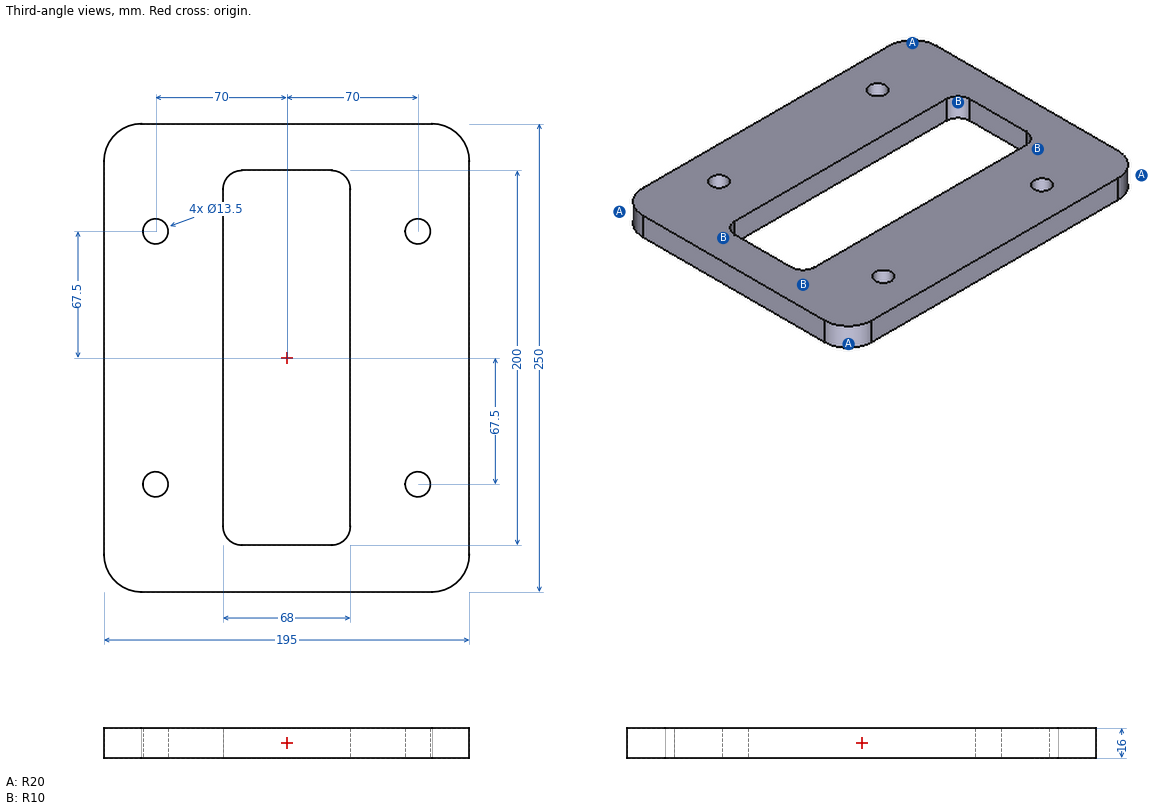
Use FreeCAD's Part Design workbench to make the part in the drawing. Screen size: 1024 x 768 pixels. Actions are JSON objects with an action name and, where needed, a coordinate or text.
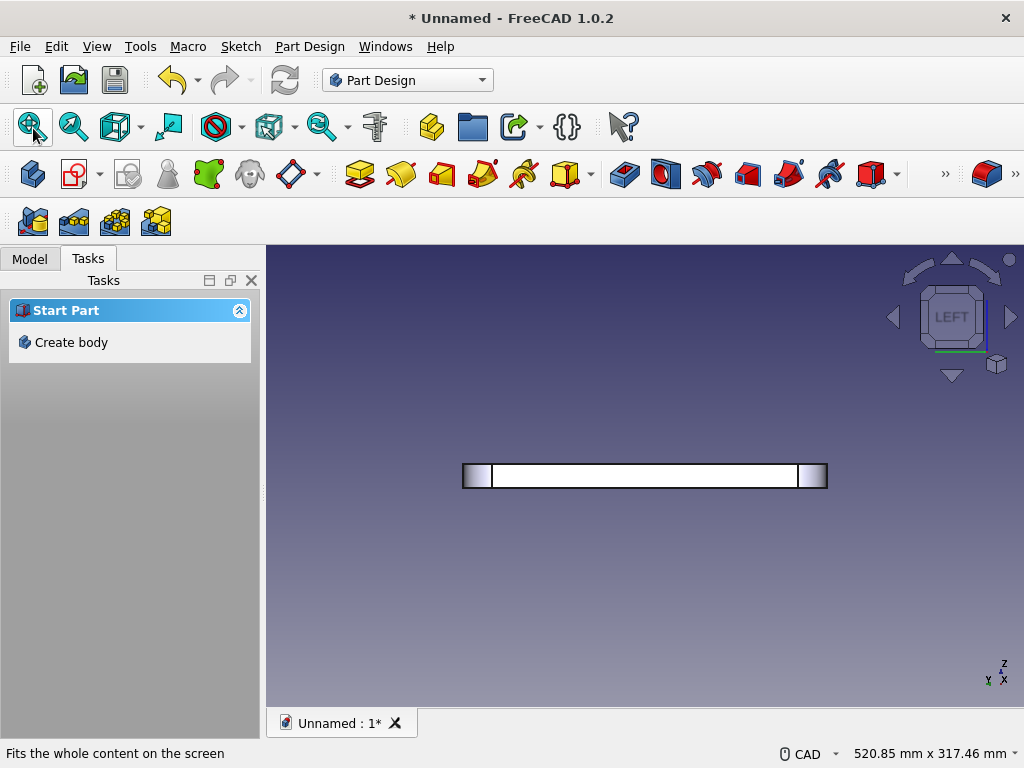
{"action": "key", "text": "v 3"}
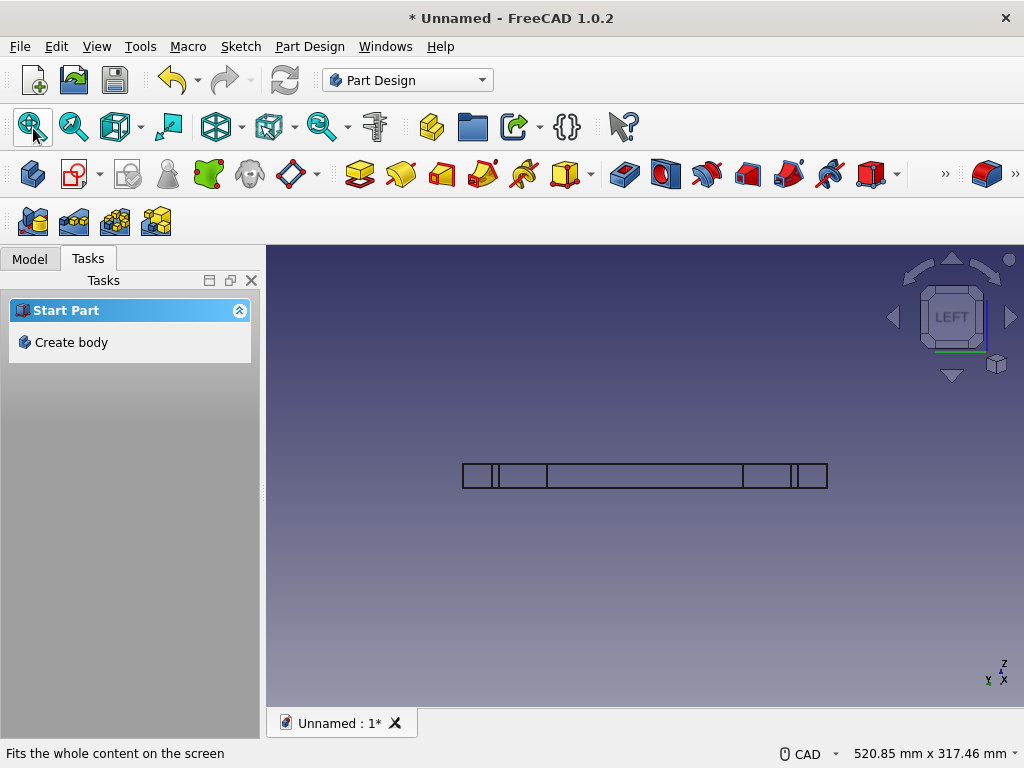
{"action": "key", "text": "0"}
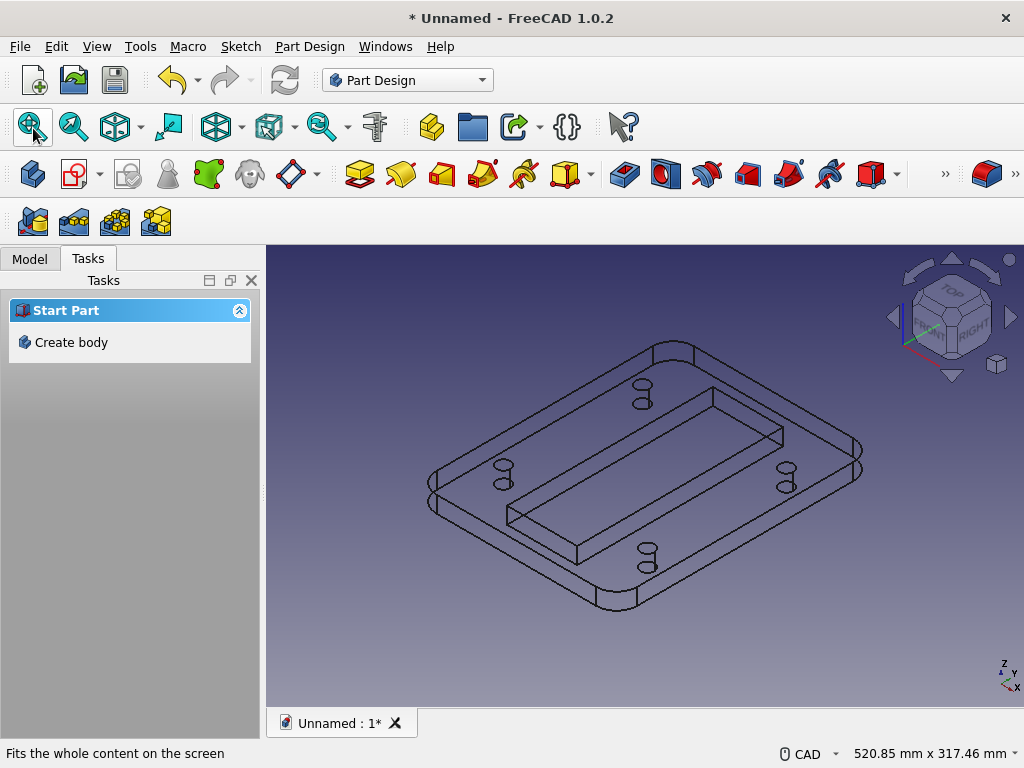
{"action": "left_click", "coordinate": [713, 395]}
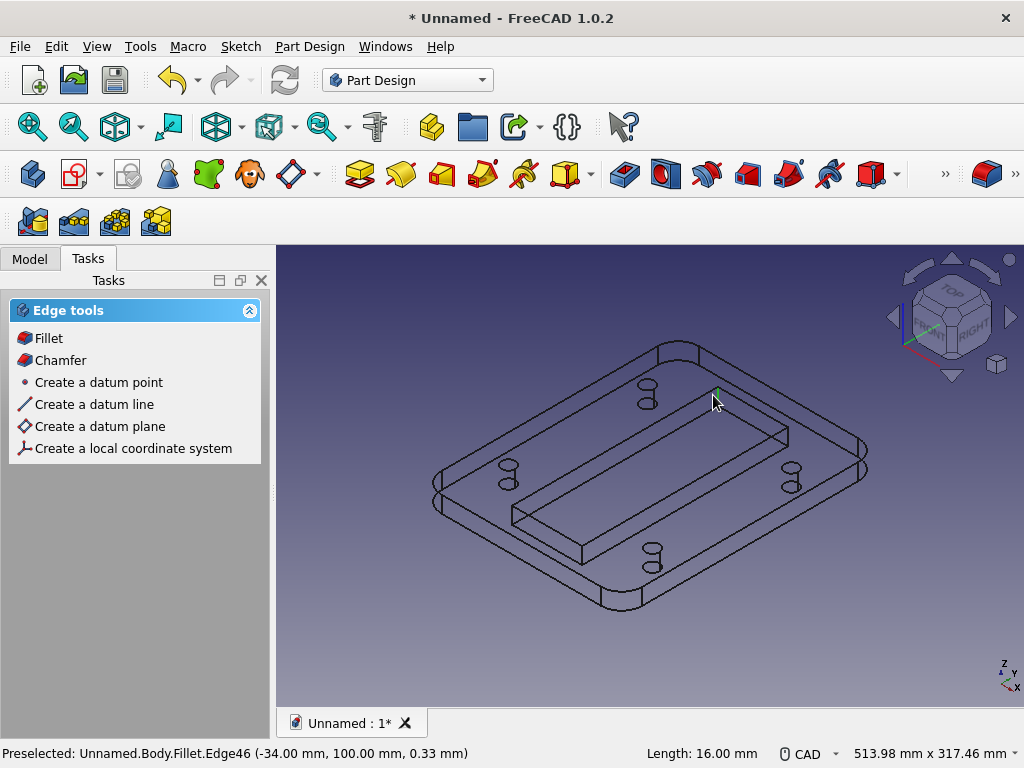
{"action": "left_click", "coordinate": [512, 514], "text": "ctrl"}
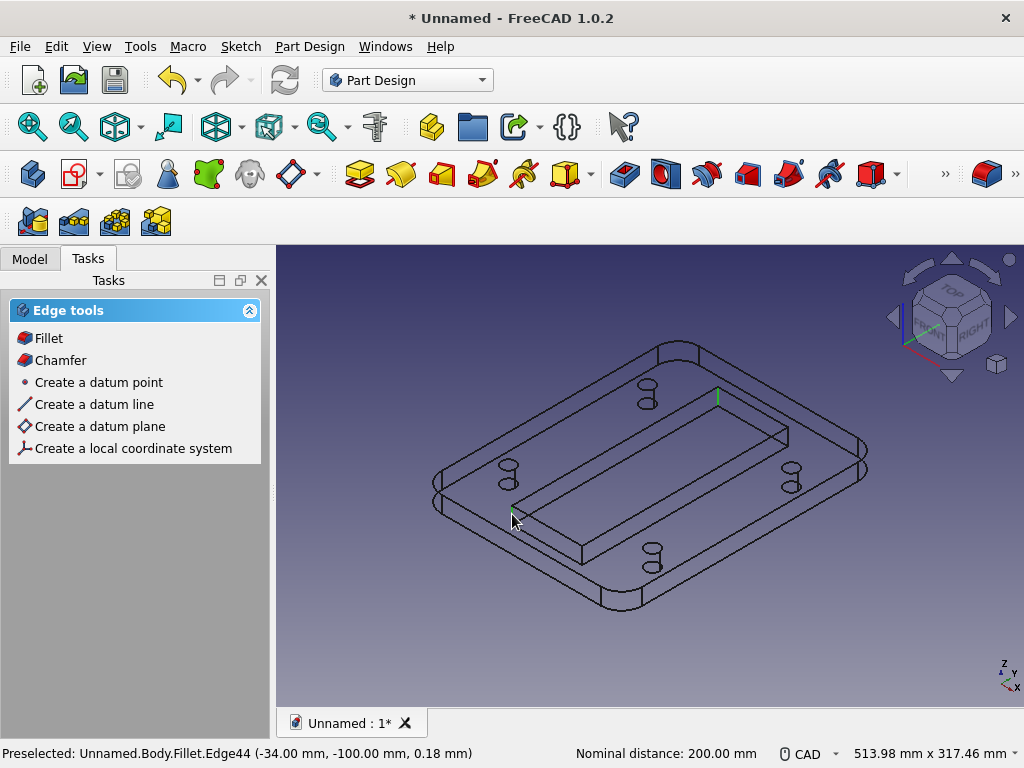
{"action": "left_click", "coordinate": [582, 555], "text": "ctrl"}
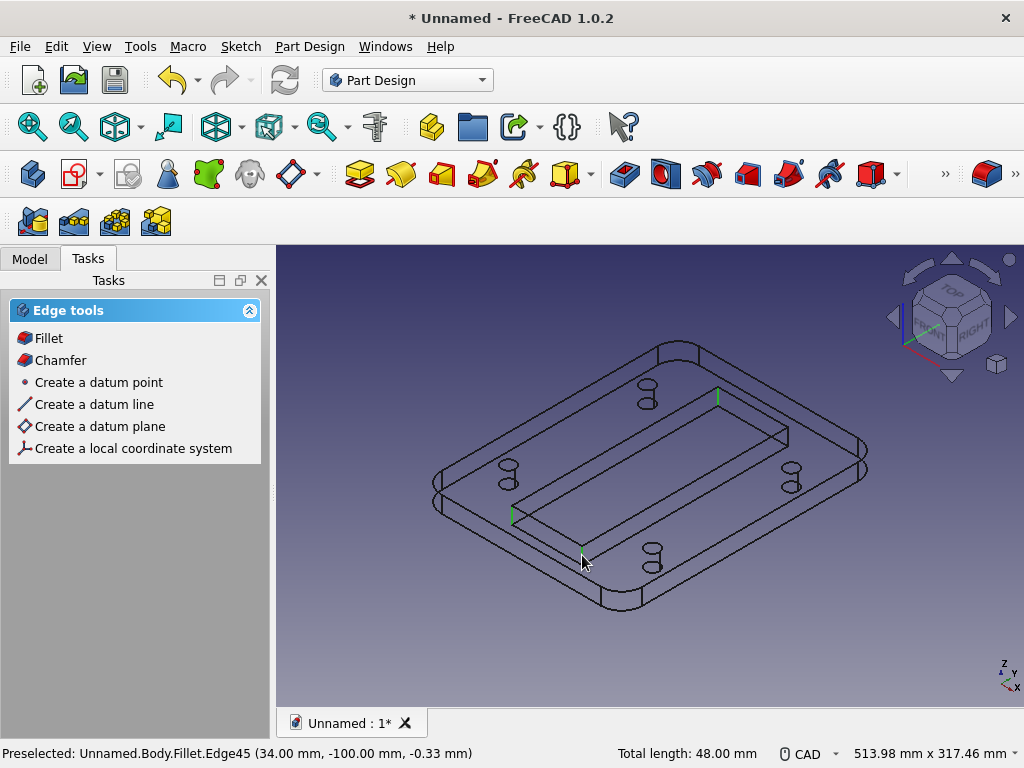
{"action": "left_click", "coordinate": [788, 436], "text": "ctrl"}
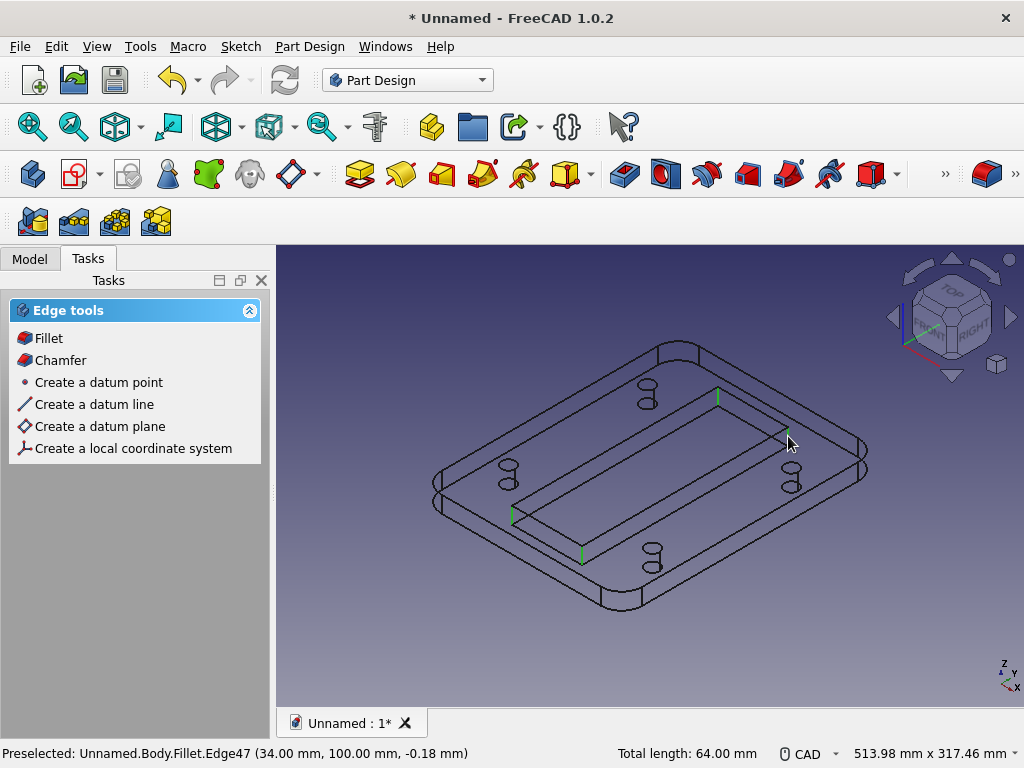
{"action": "key", "text": "v 1"}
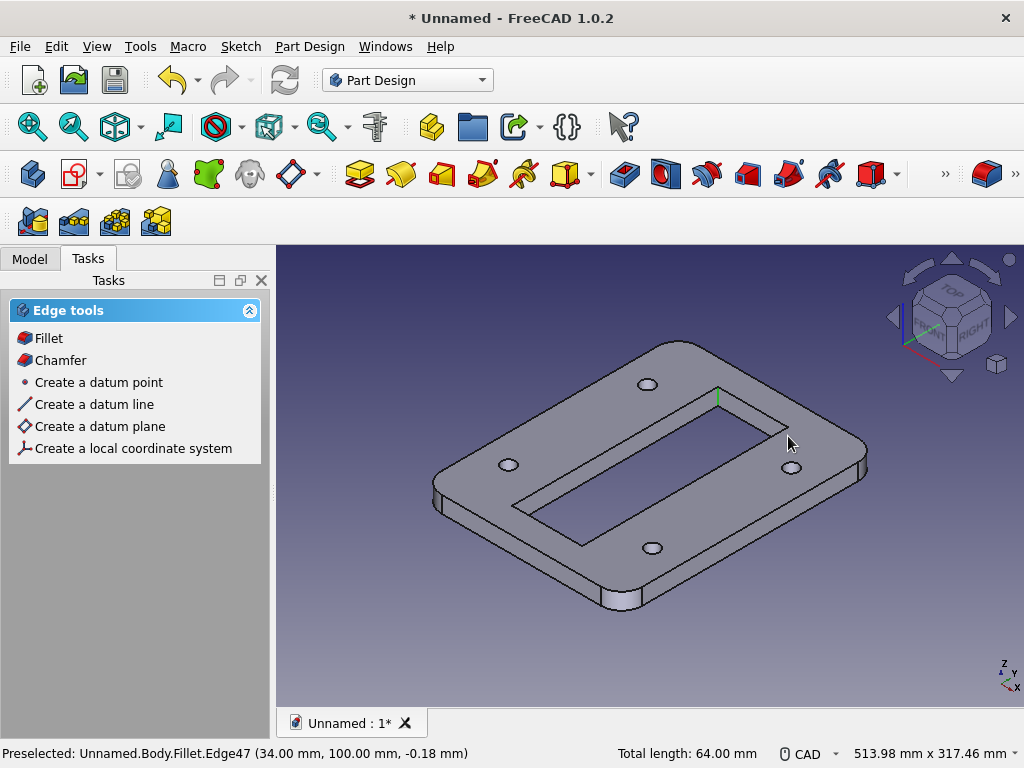
{"action": "left_click", "coordinate": [987, 174]}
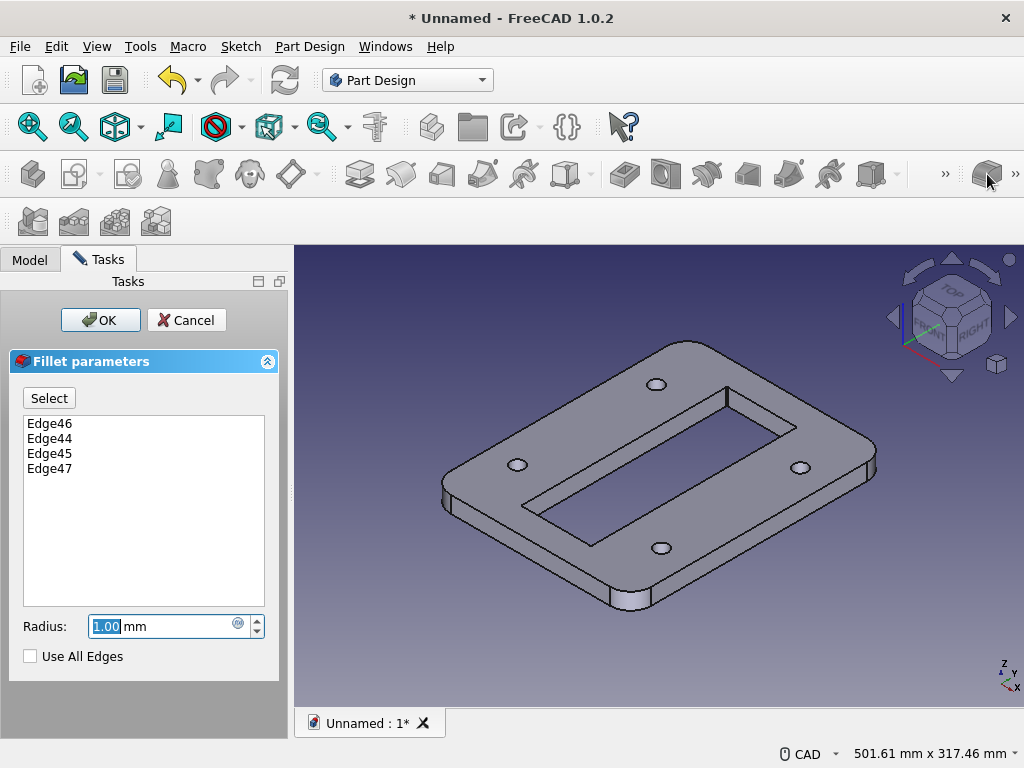
{"action": "type", "text": "10"}
{"action": "key", "text": "Tab"}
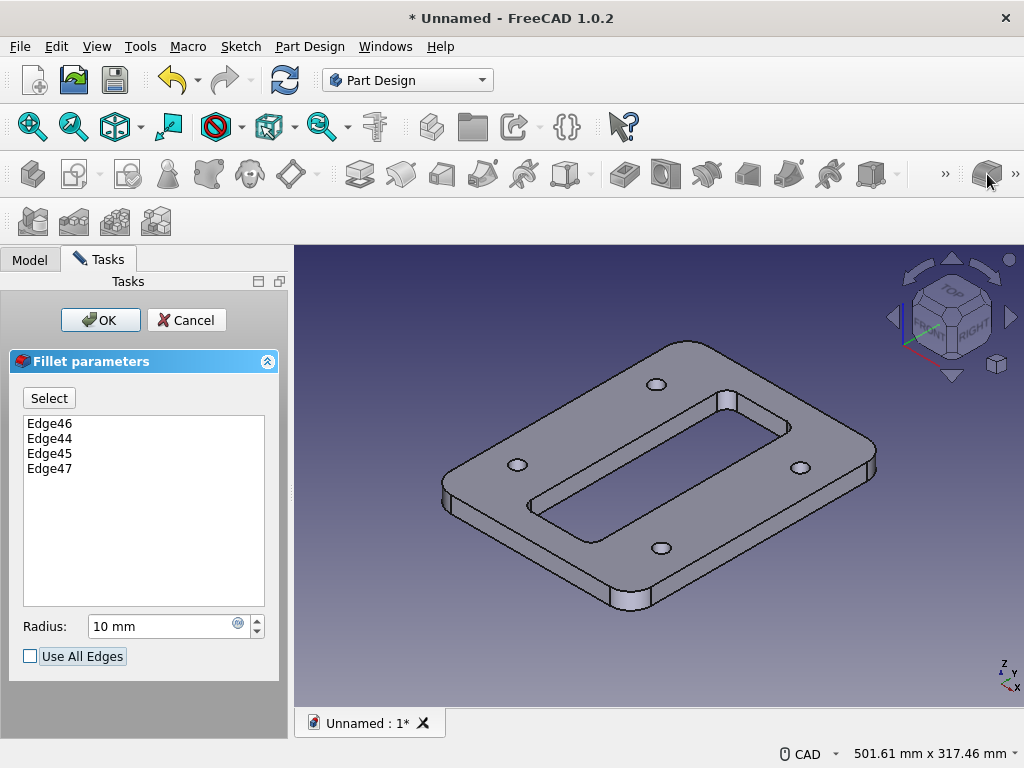
{"action": "left_click", "coordinate": [101, 320]}